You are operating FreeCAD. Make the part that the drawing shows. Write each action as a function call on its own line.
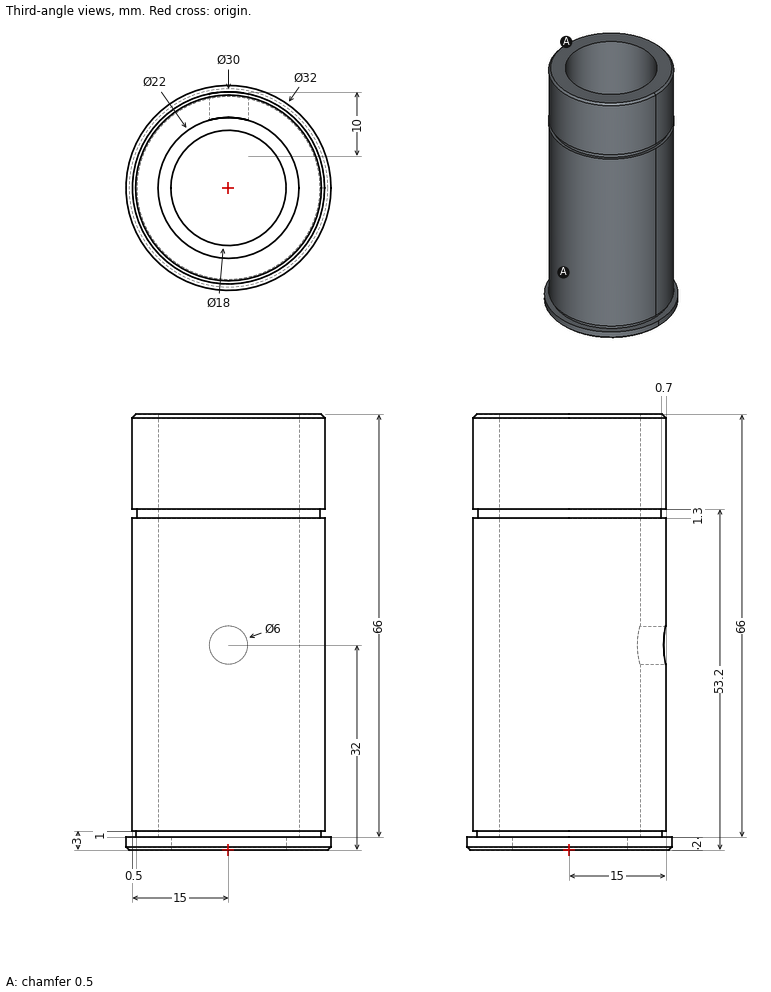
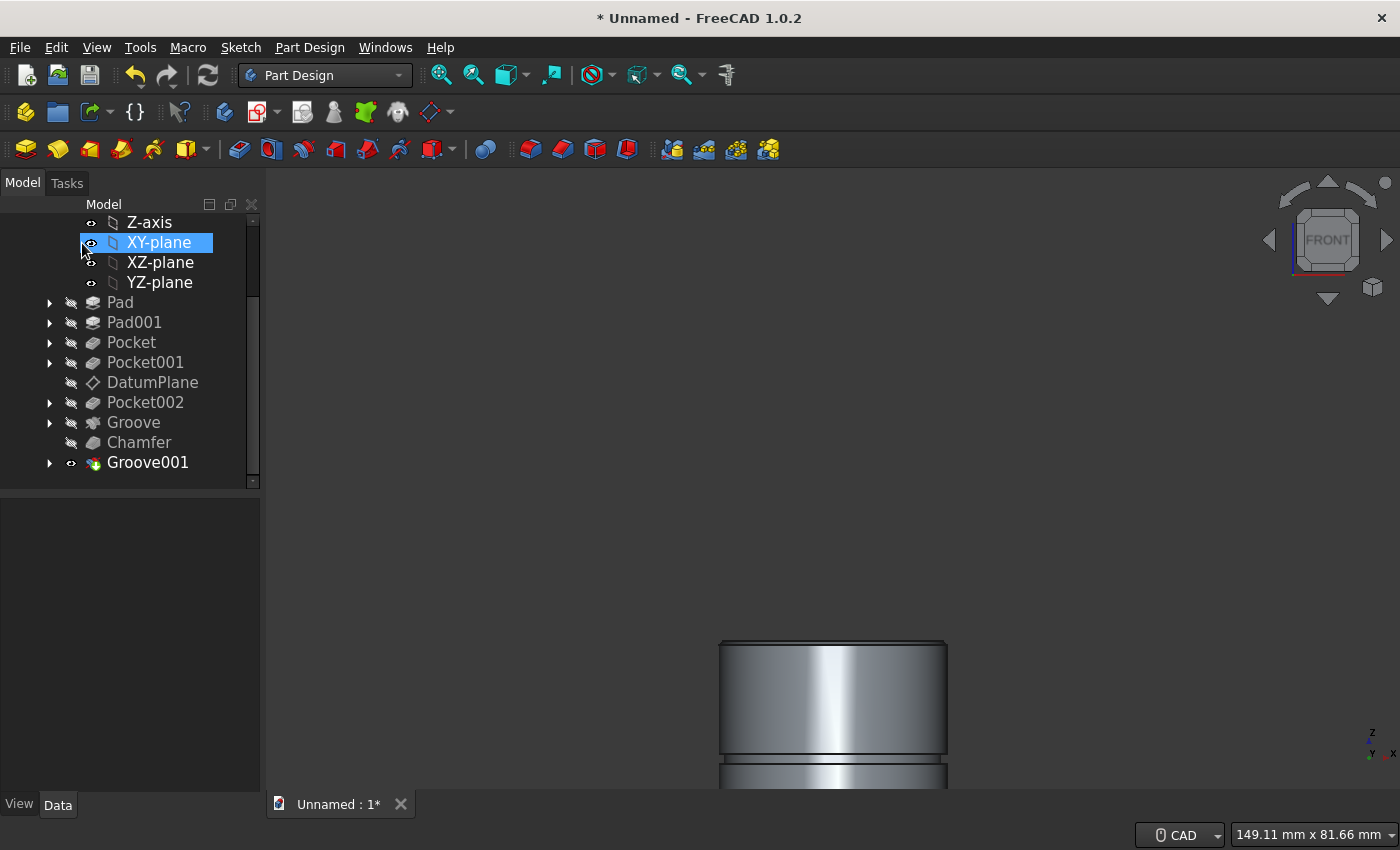
key(0)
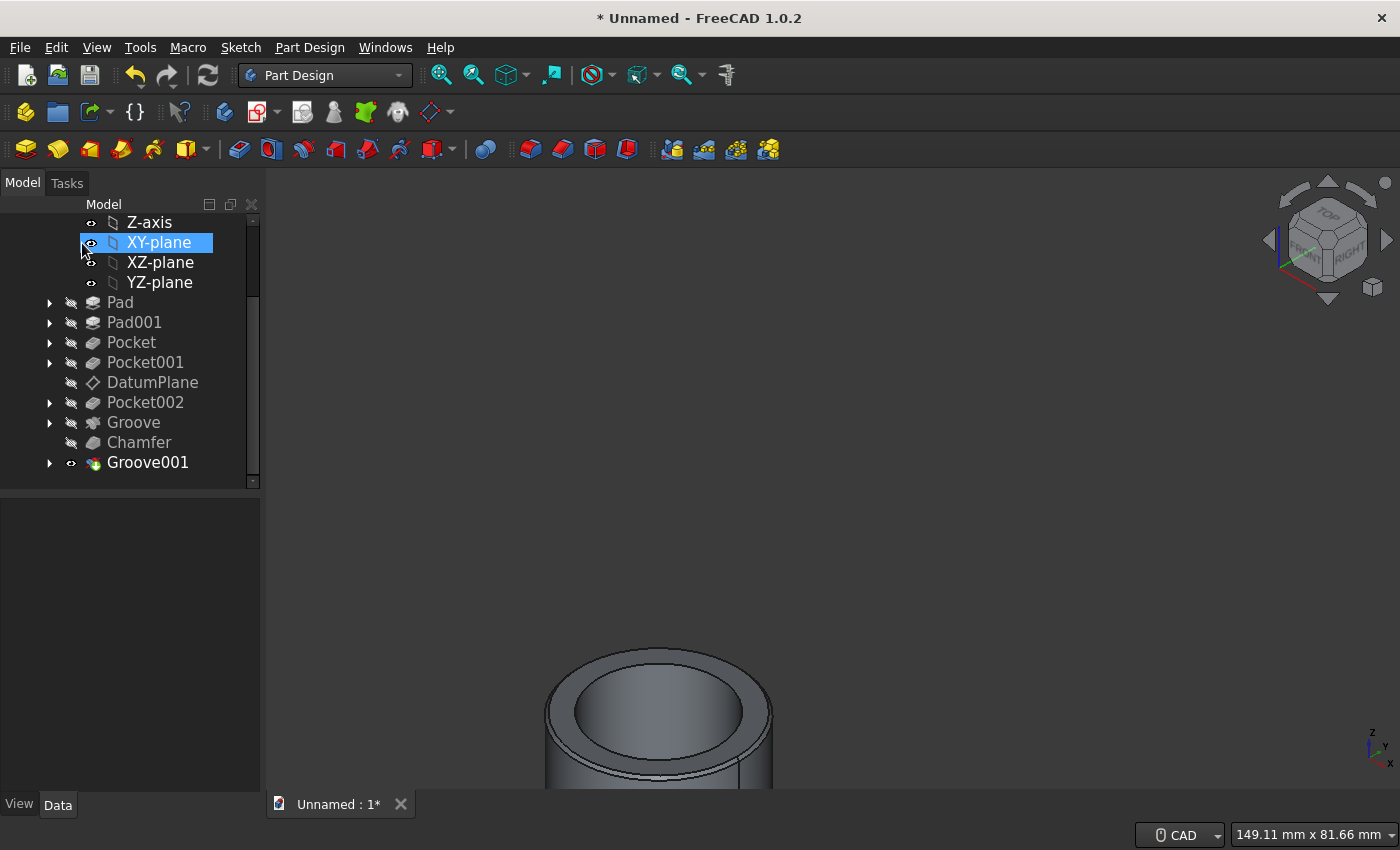
key(v)
key(f)